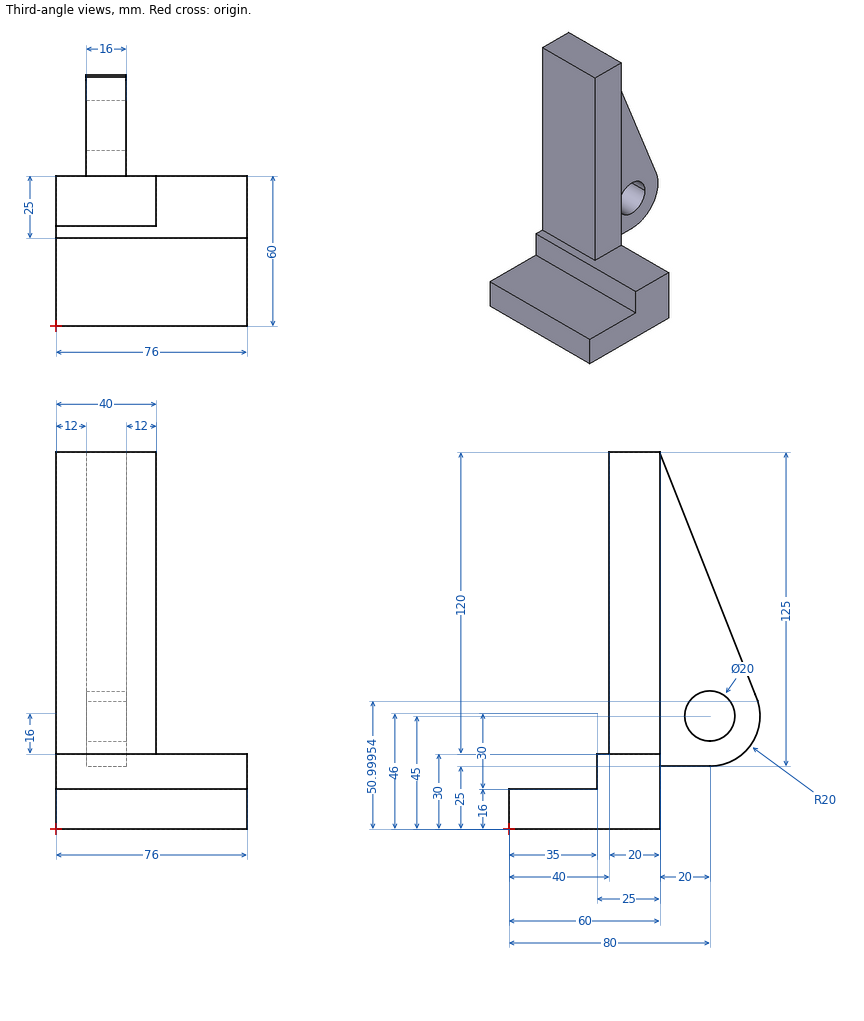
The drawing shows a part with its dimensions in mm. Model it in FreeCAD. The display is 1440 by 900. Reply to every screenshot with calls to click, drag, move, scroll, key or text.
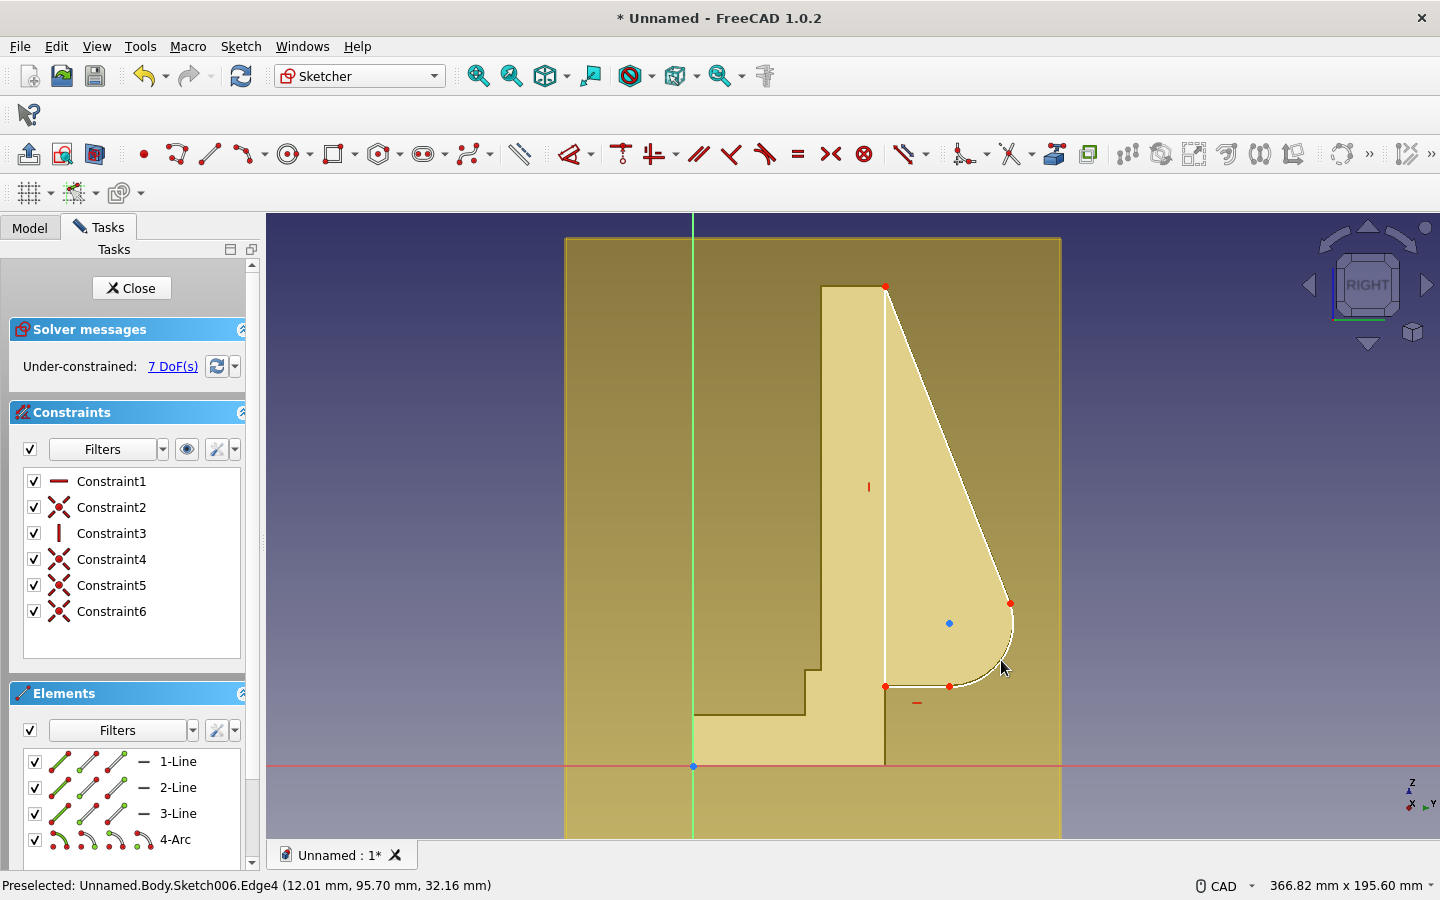
click(930, 687)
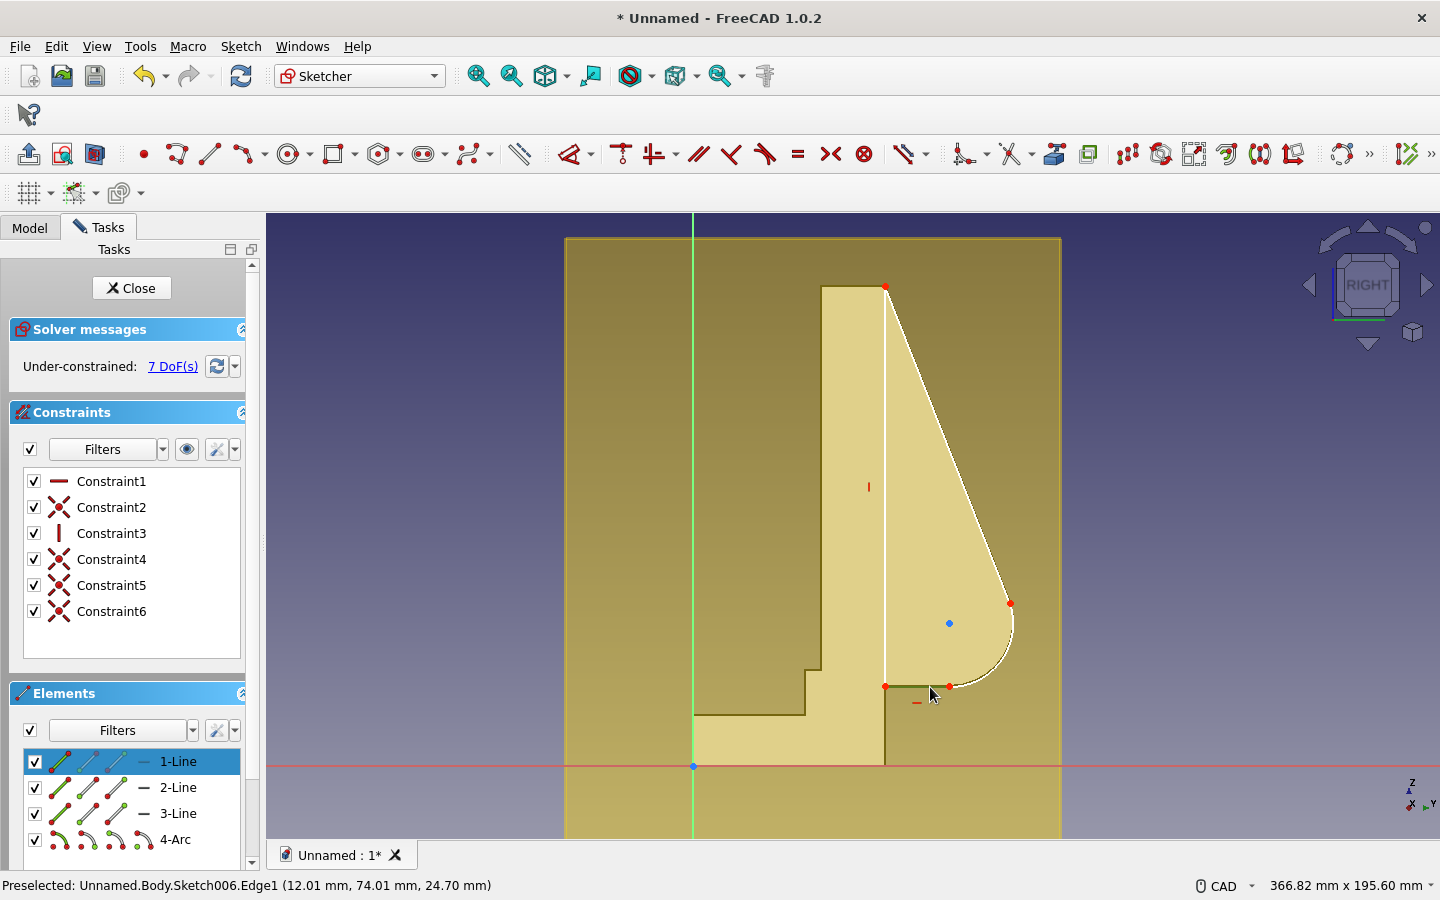
click(983, 677)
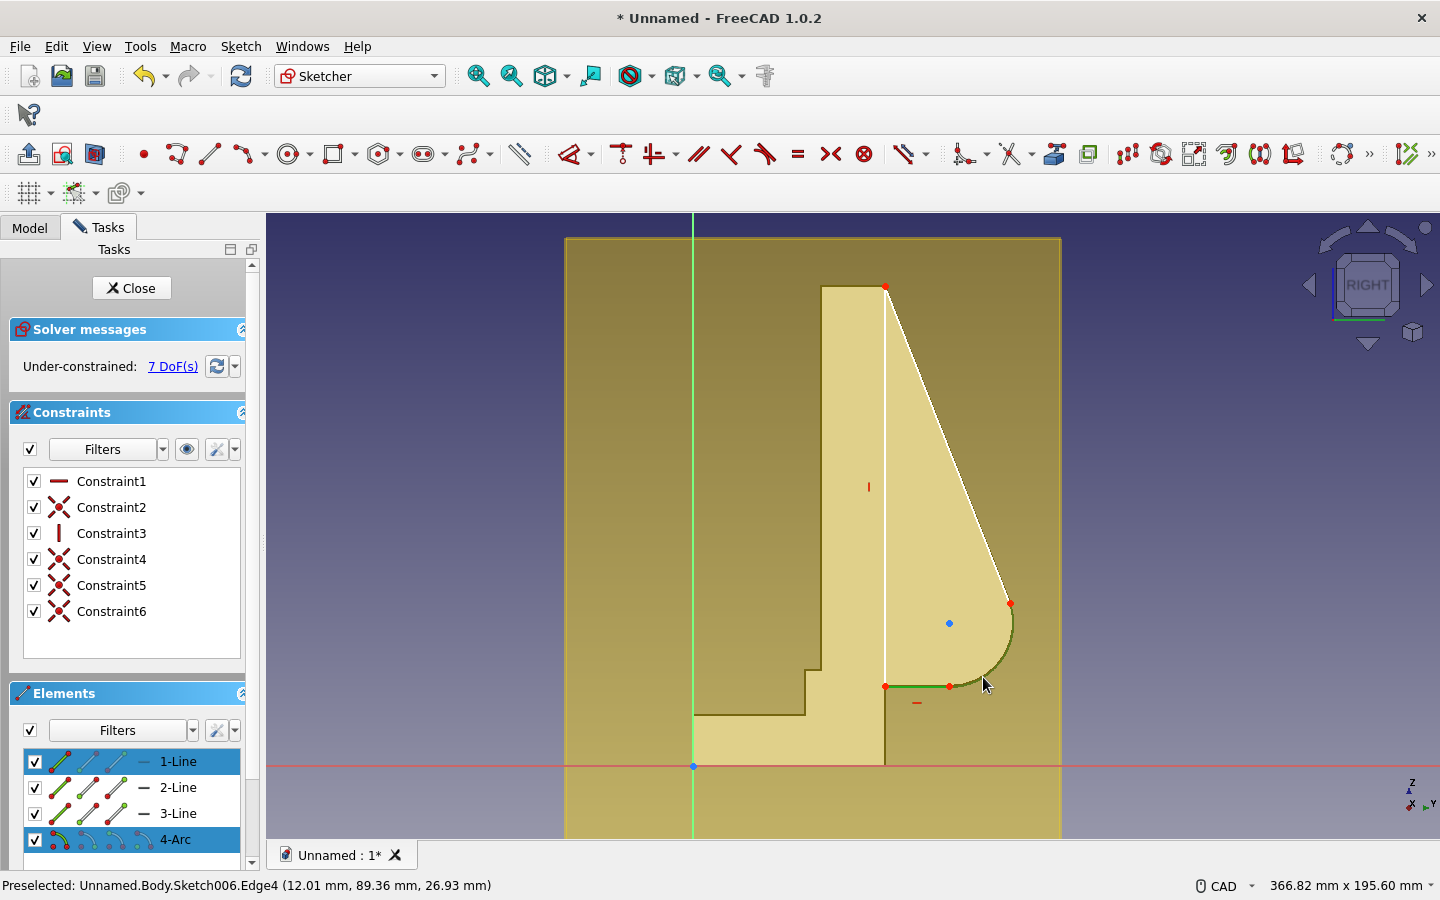
click(765, 154)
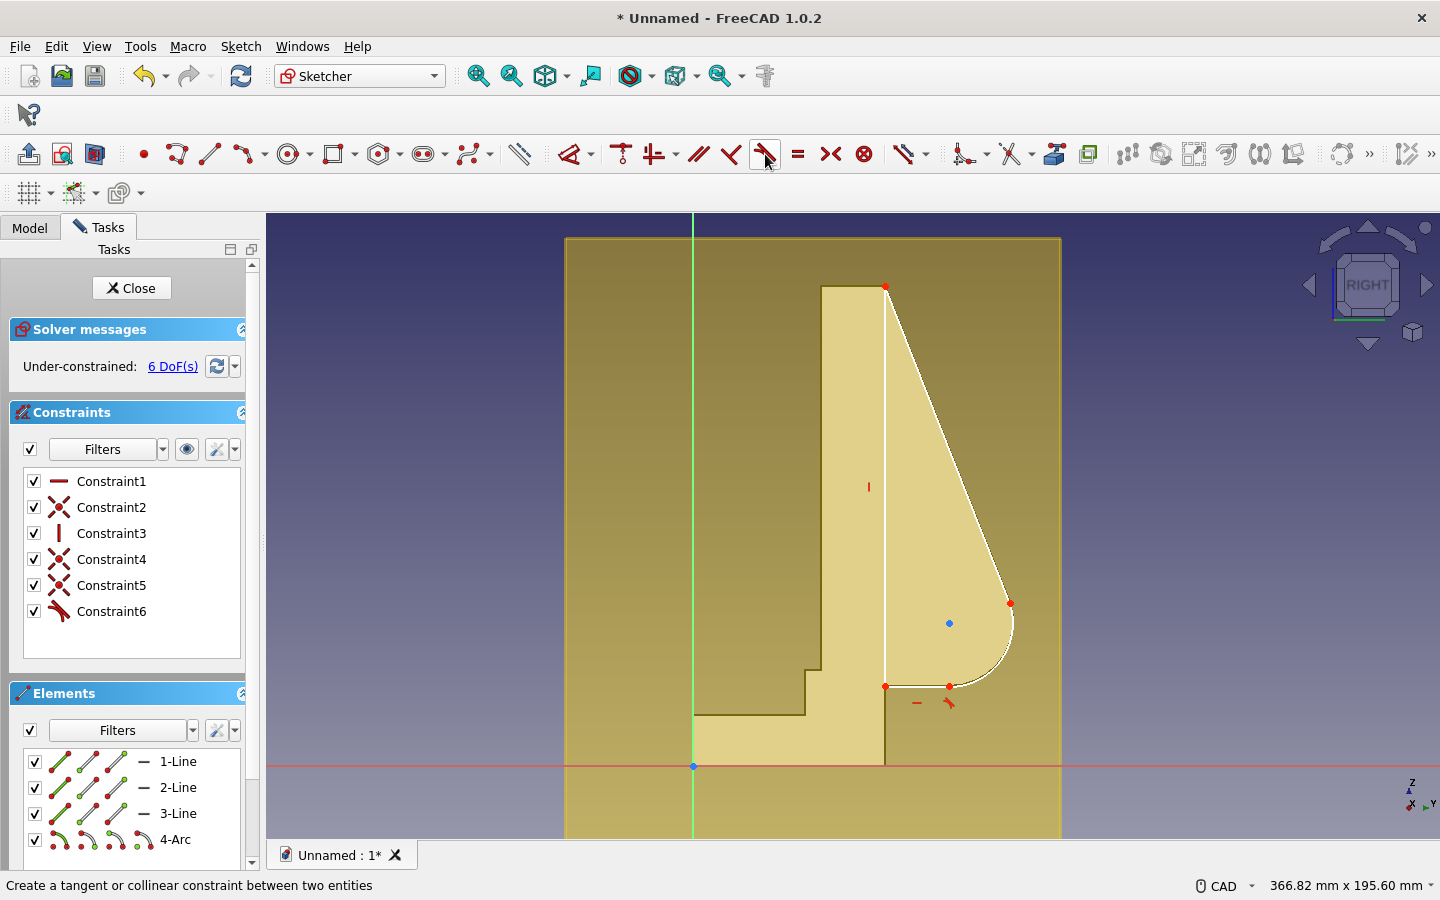
key(d)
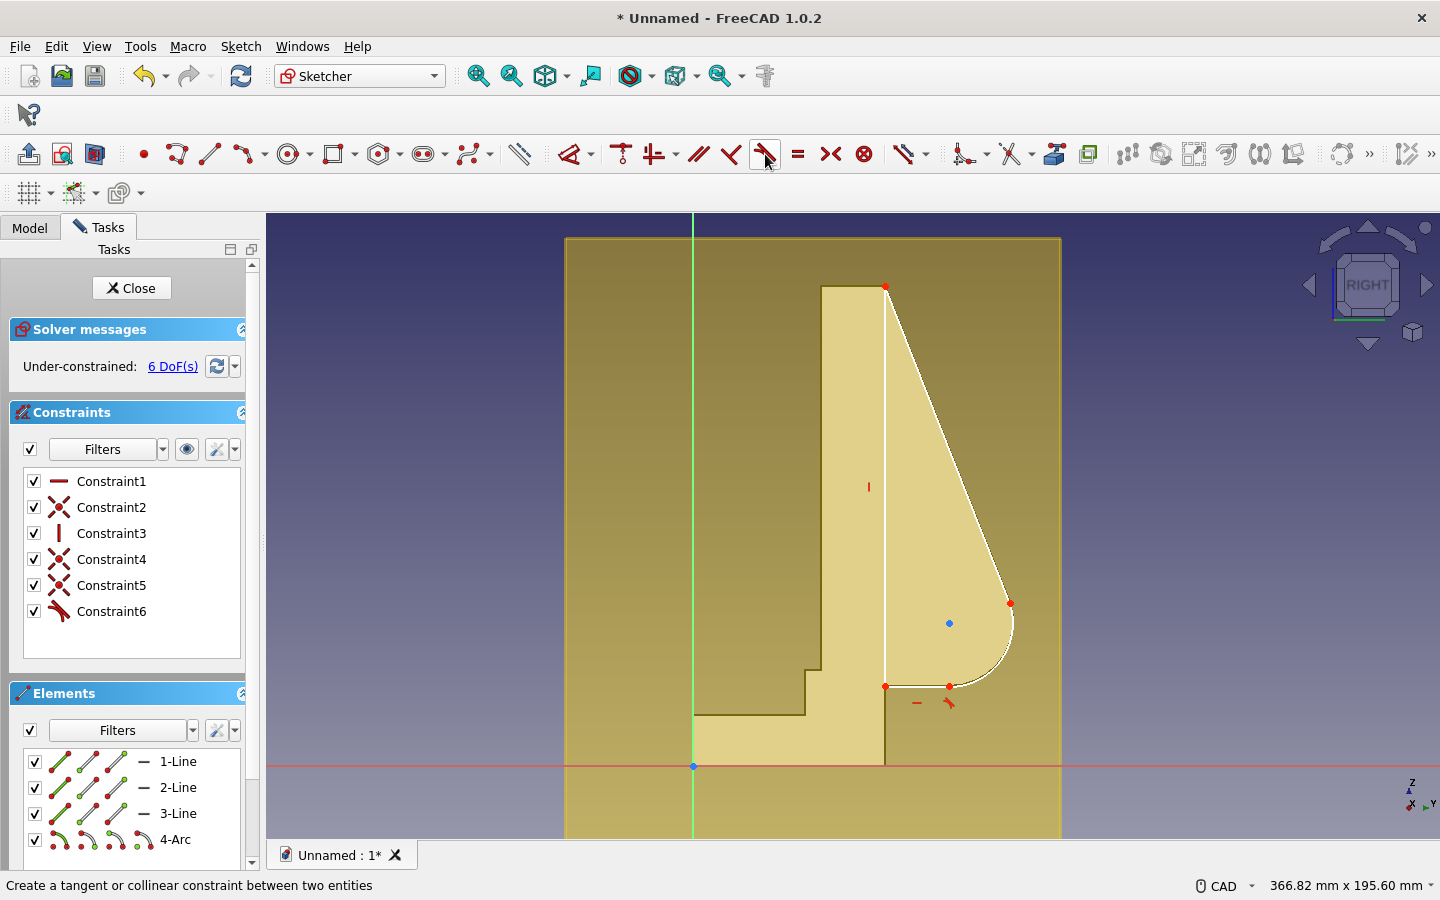
click(983, 677)
click(1000, 704)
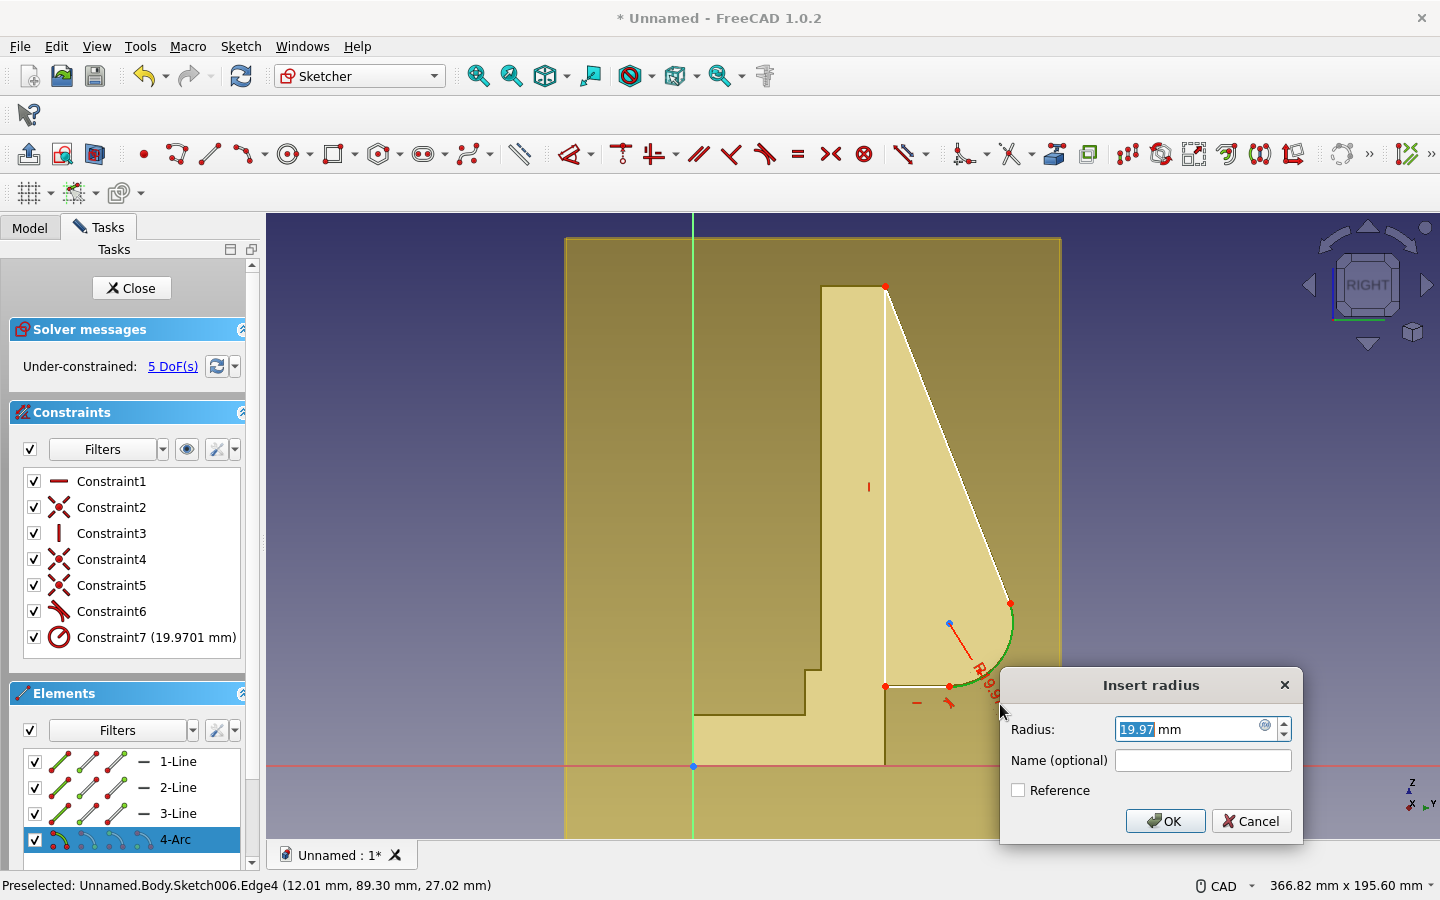
text(20)
key(Return)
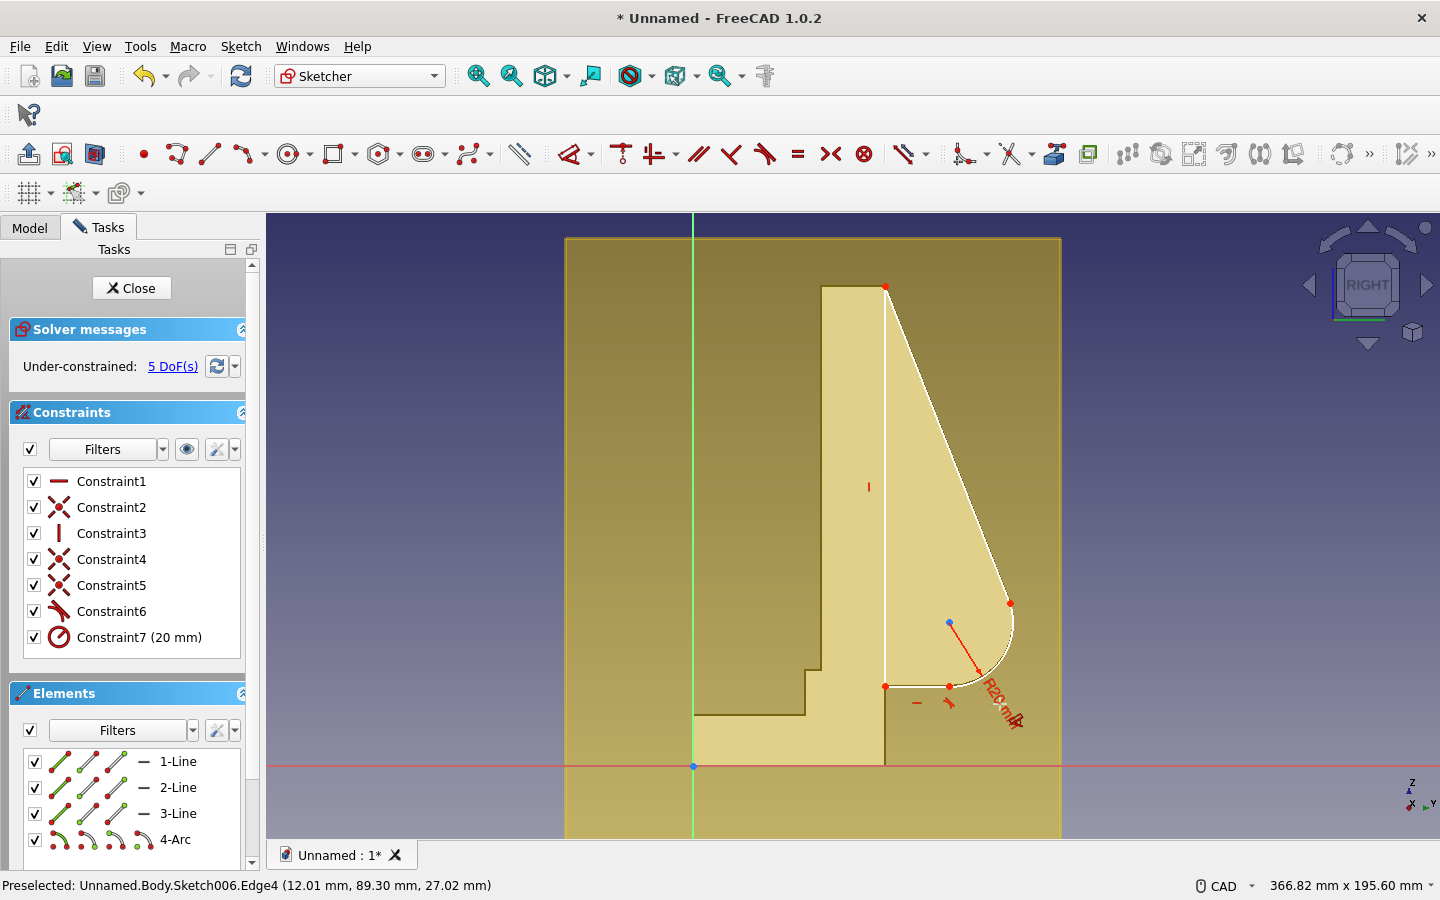
click(930, 687)
click(917, 721)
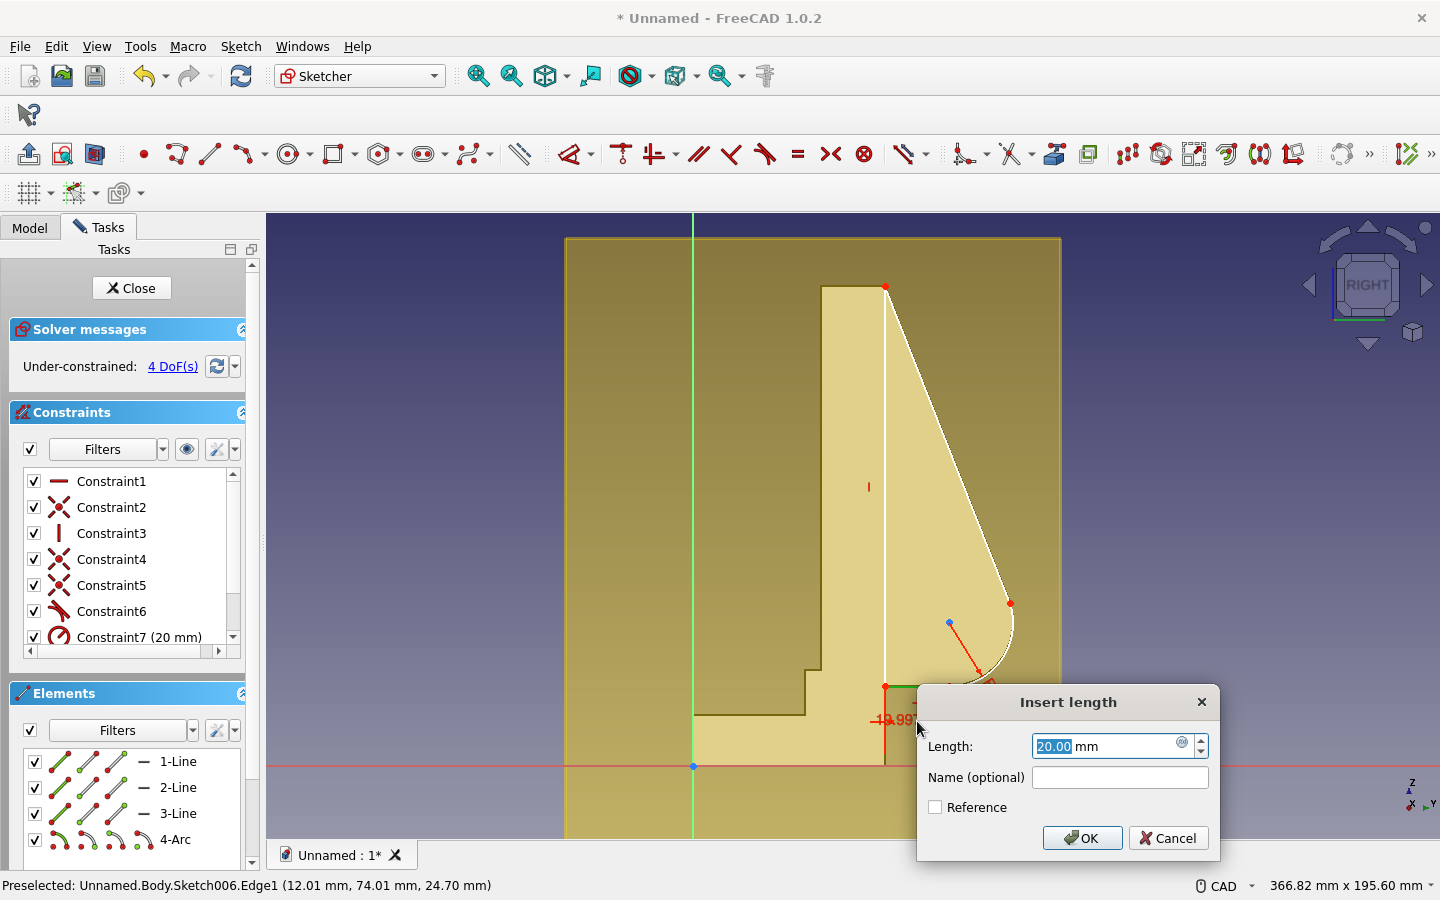
text(20)
key(Return)